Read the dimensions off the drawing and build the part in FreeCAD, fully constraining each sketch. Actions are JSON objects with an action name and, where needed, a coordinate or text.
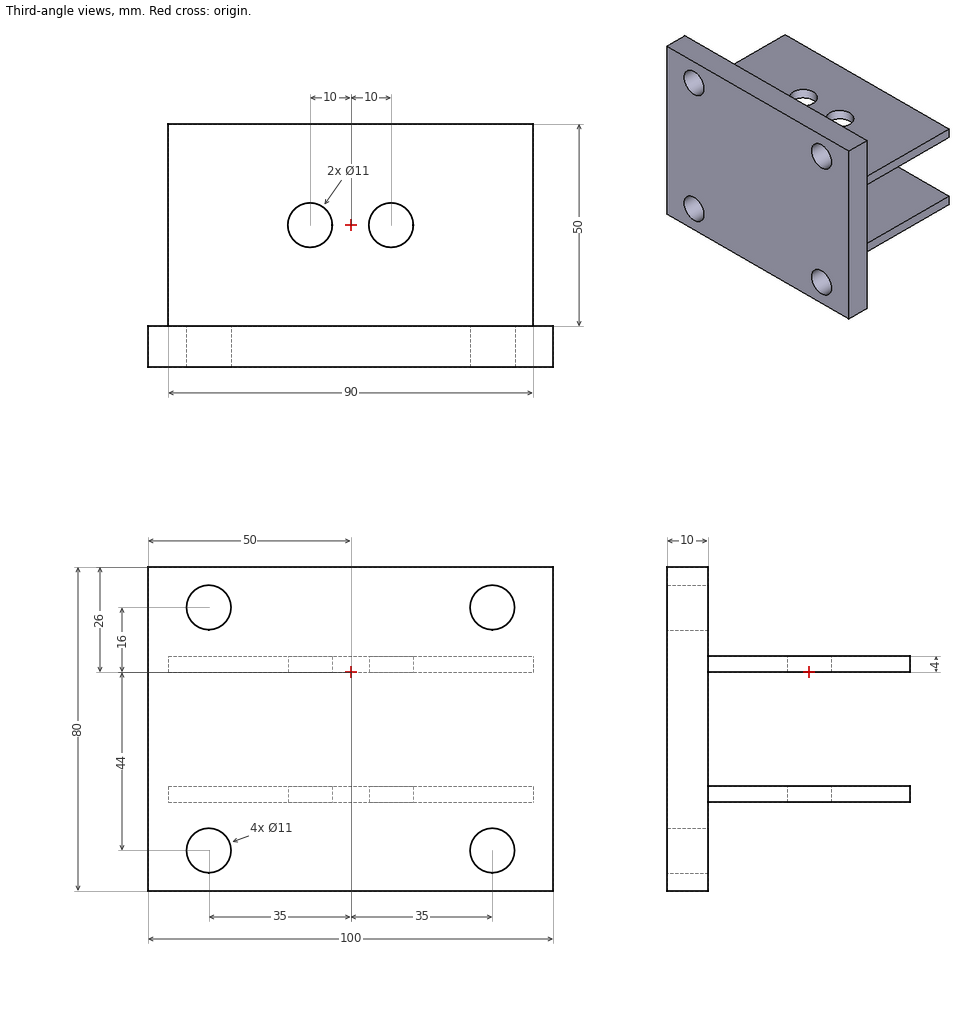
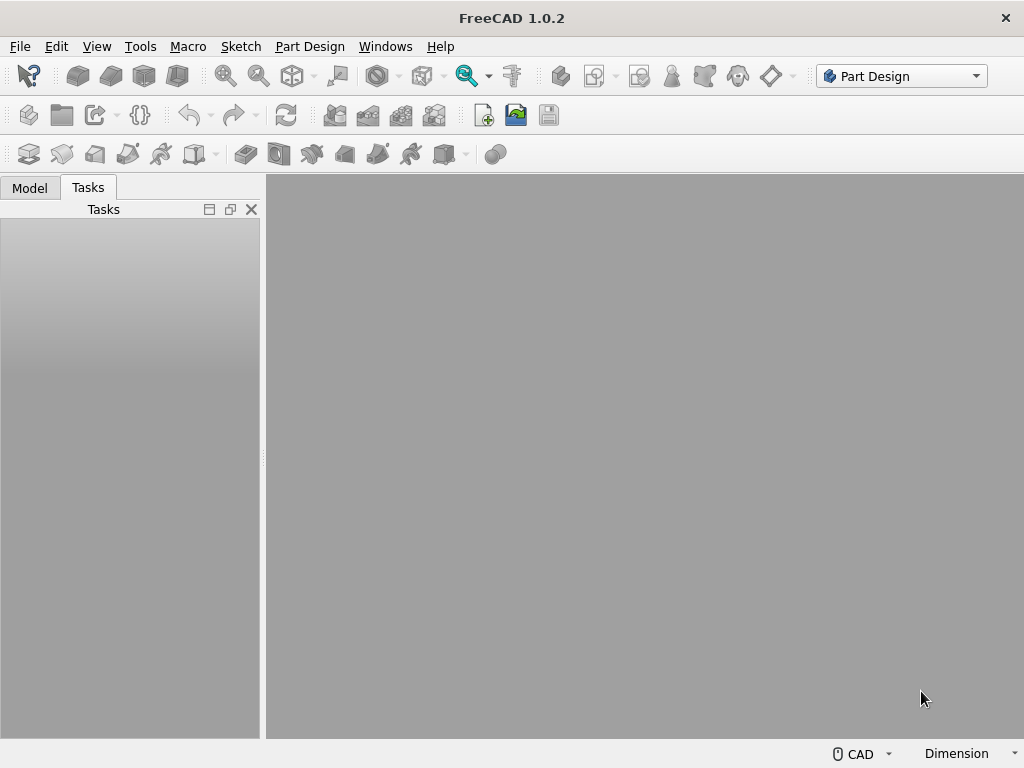
{"action": "key", "text": "ctrl+n"}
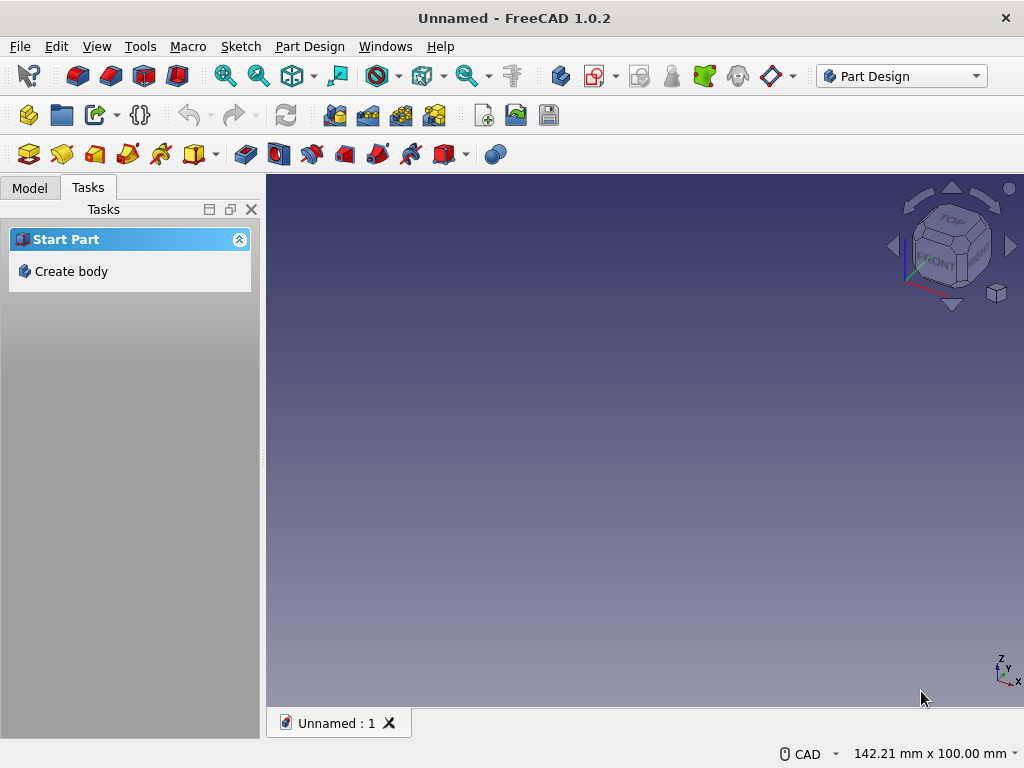
{"action": "left_click", "coordinate": [594, 76]}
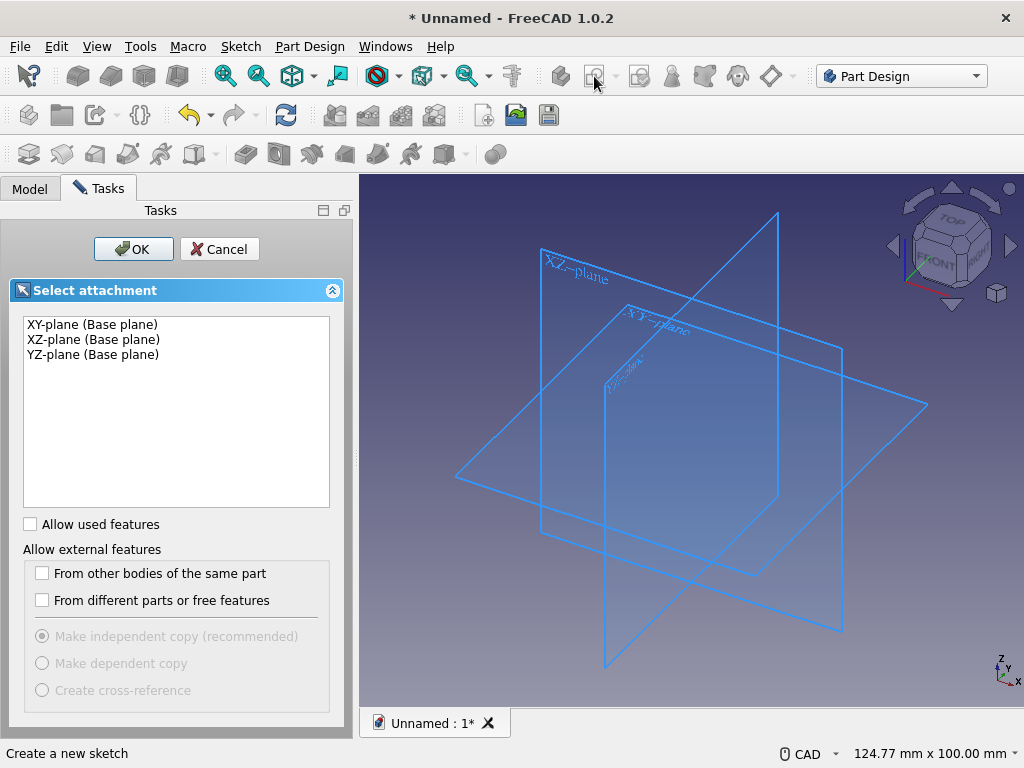
{"action": "left_click", "coordinate": [84, 324]}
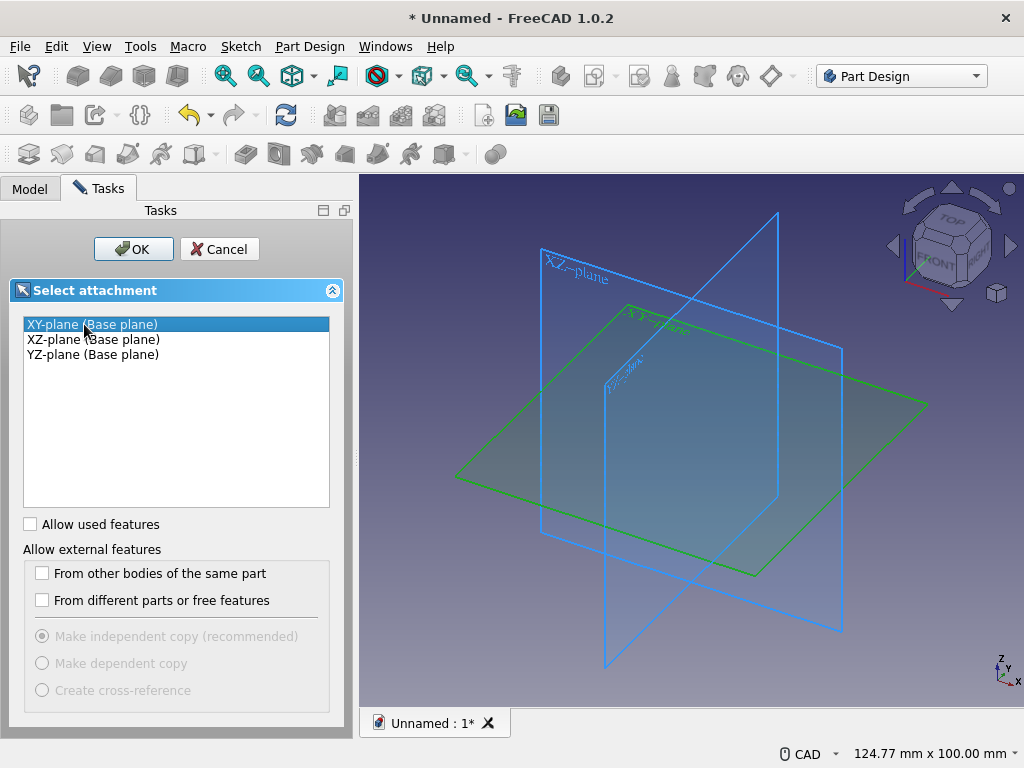
{"action": "left_click", "coordinate": [134, 249]}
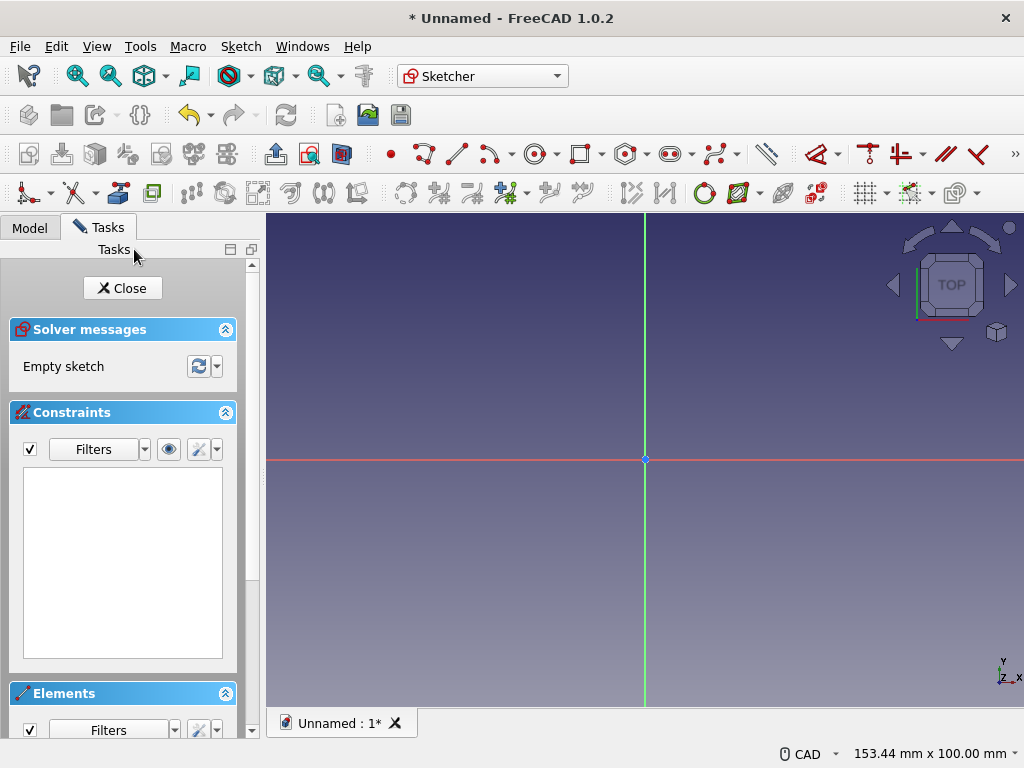
{"action": "scroll", "coordinate": [294, 460], "scroll_direction": "down", "scroll_amount": 1}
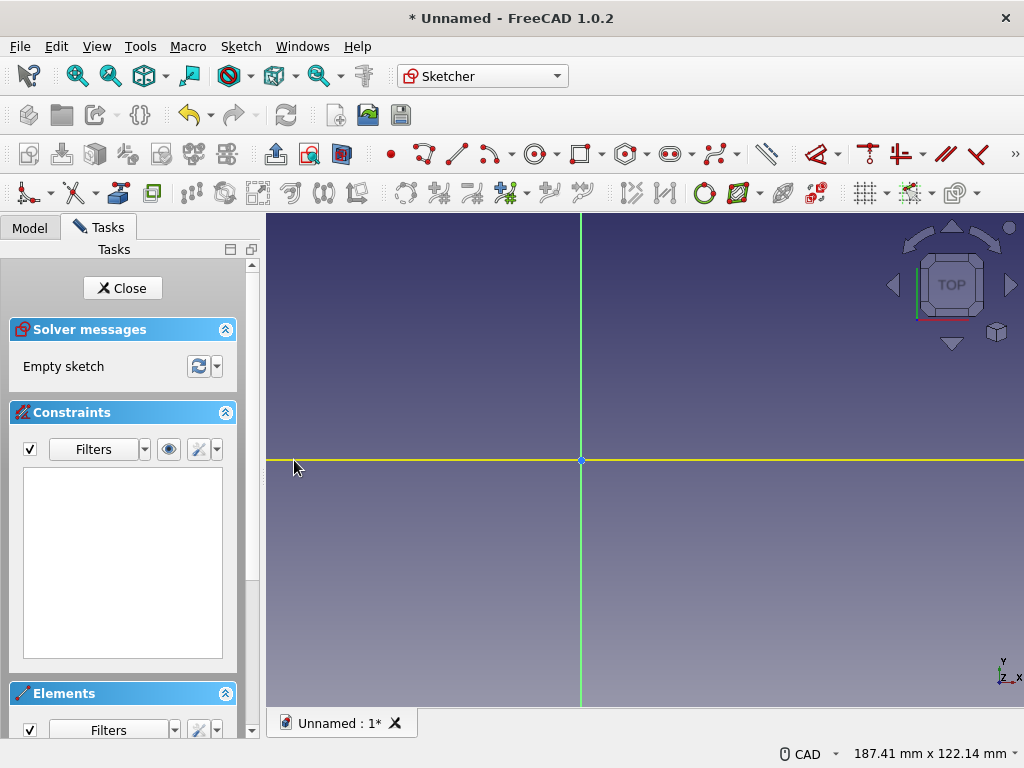
{"action": "key", "text": "g v"}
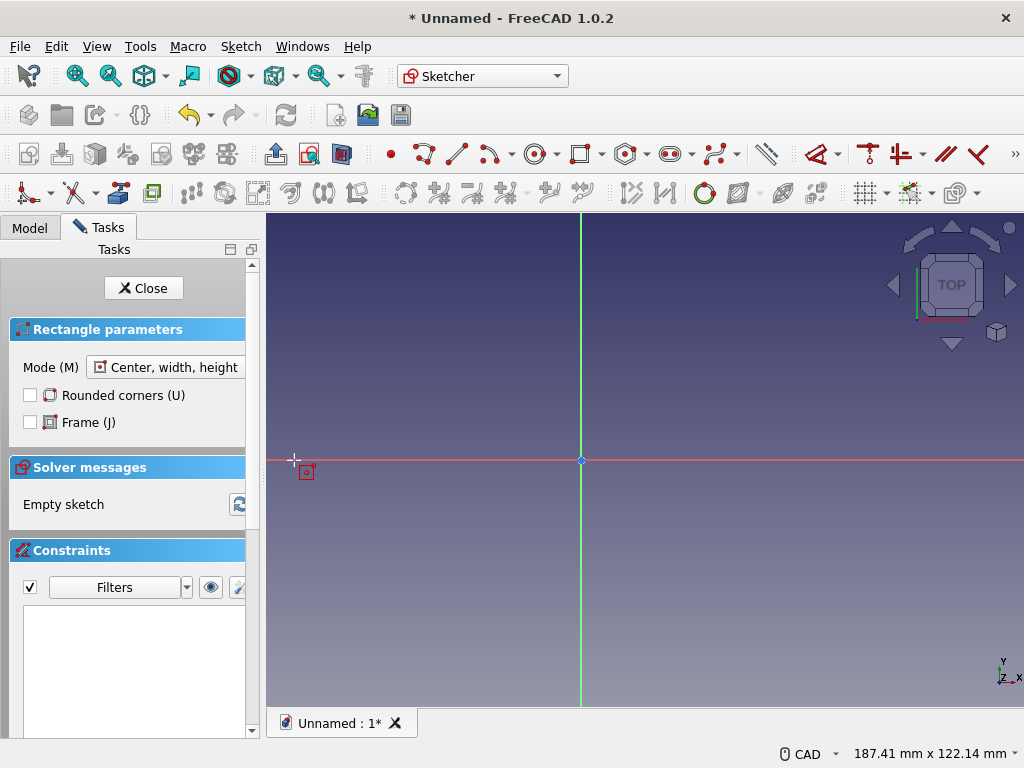
{"action": "left_click", "coordinate": [581, 460]}
{"action": "left_click", "coordinate": [763, 359]}
{"action": "key", "text": "Escape"}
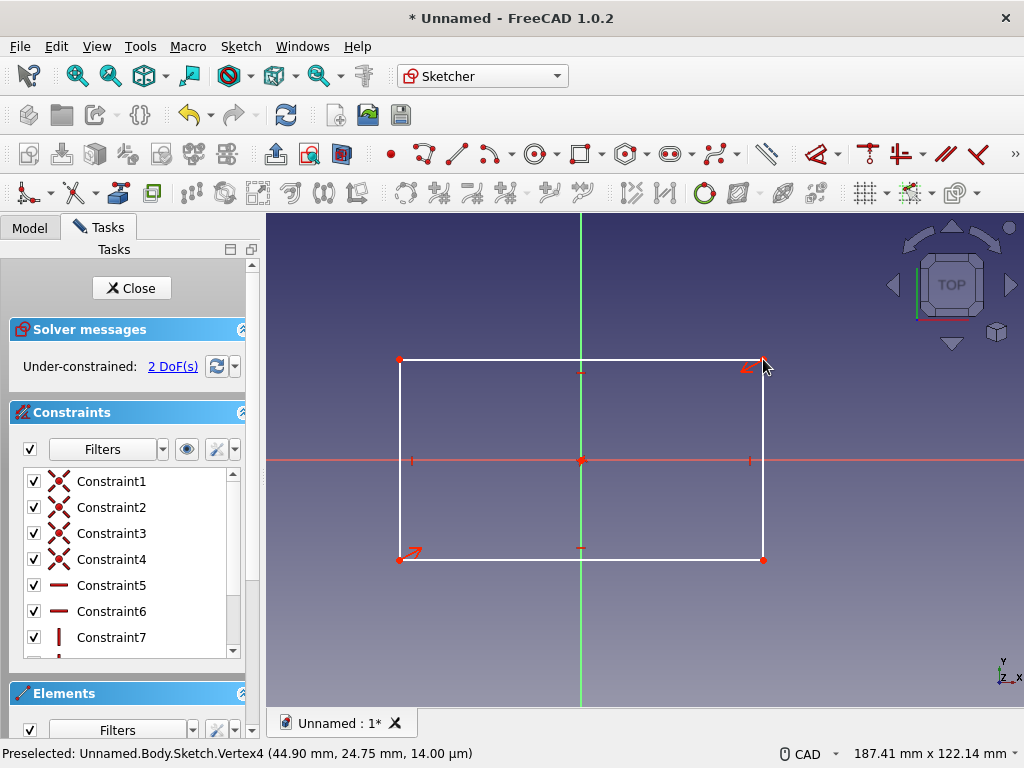
{"action": "key", "text": "d"}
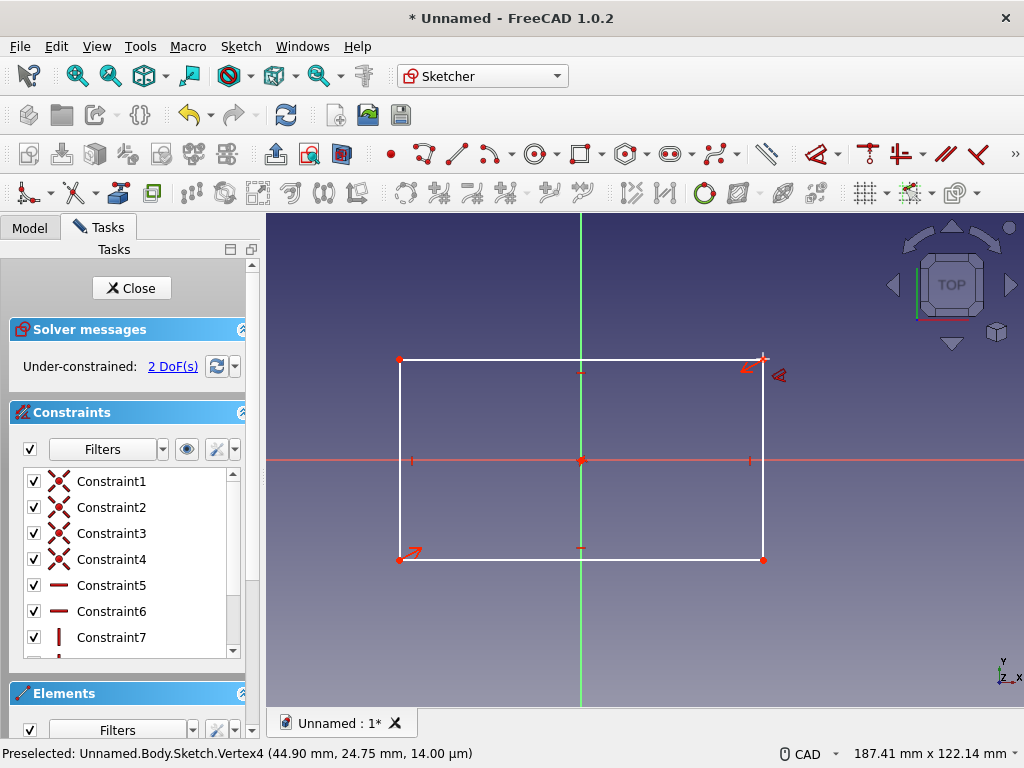
{"action": "left_click", "coordinate": [509, 560]}
{"action": "left_click", "coordinate": [498, 594]}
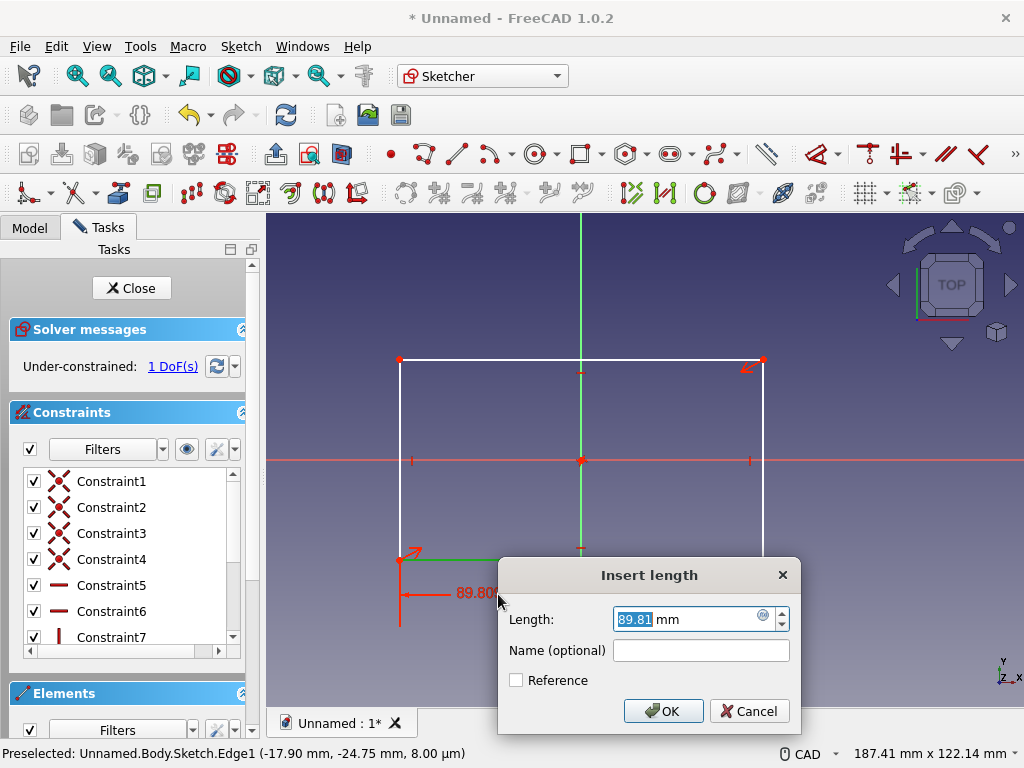
{"action": "type", "text": "90"}
{"action": "key", "text": "Return"}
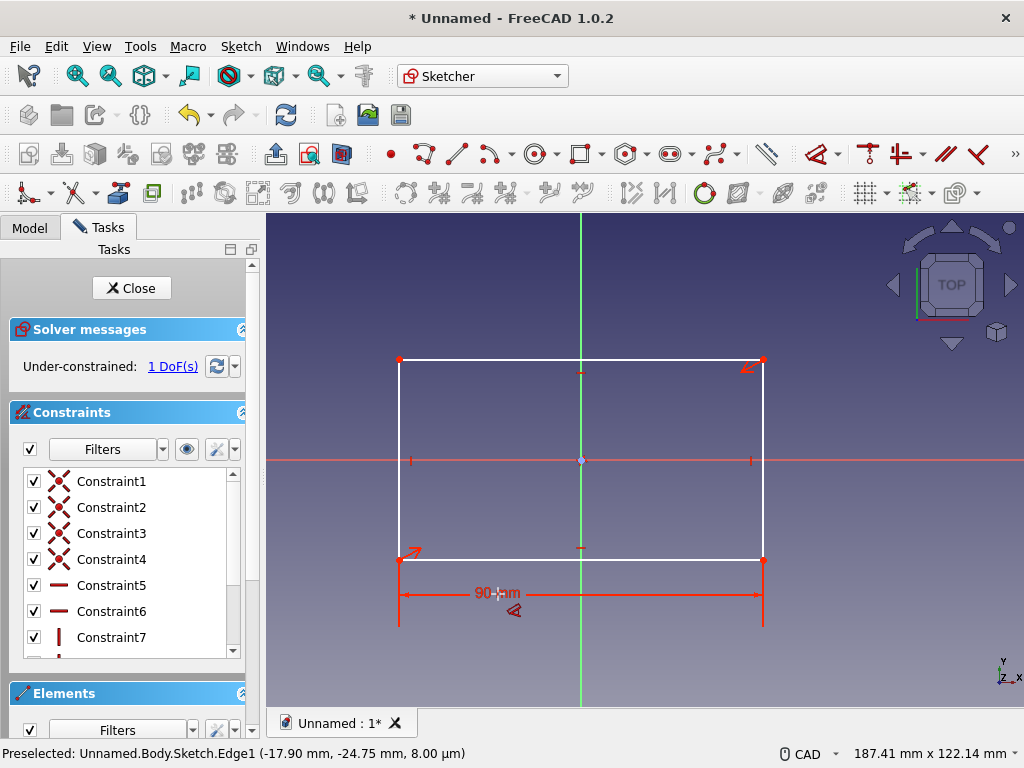
{"action": "left_click", "coordinate": [763, 500]}
{"action": "left_click", "coordinate": [797, 414]}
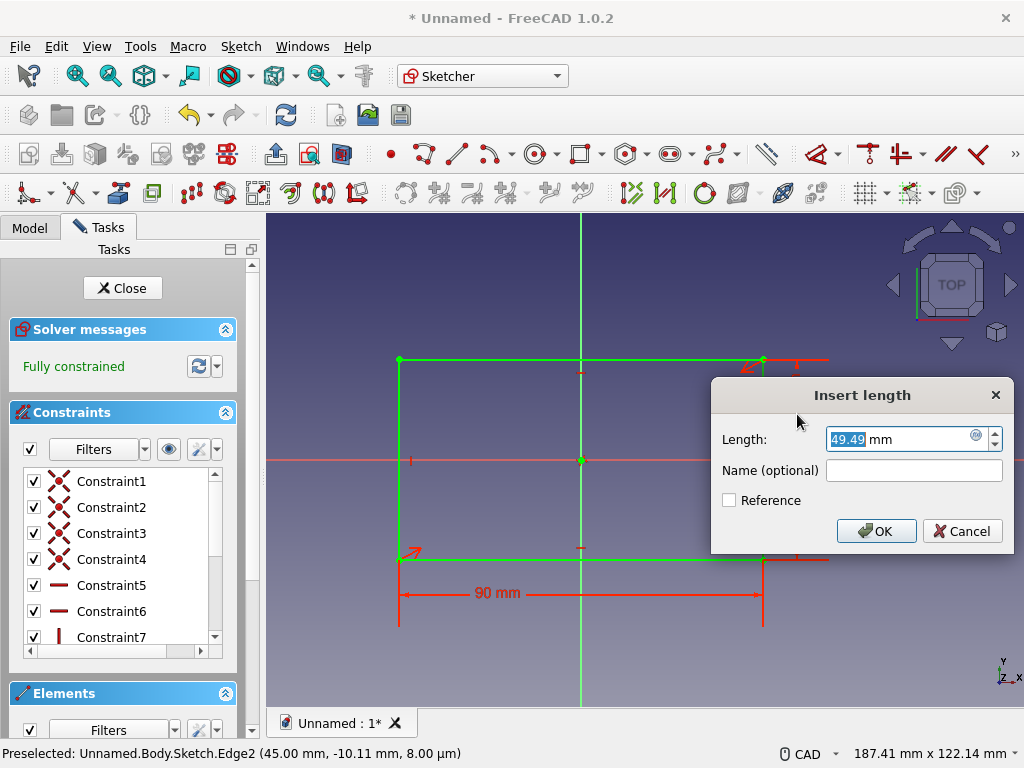
{"action": "type", "text": "50"}
{"action": "key", "text": "Return"}
{"action": "key", "text": "Escape"}